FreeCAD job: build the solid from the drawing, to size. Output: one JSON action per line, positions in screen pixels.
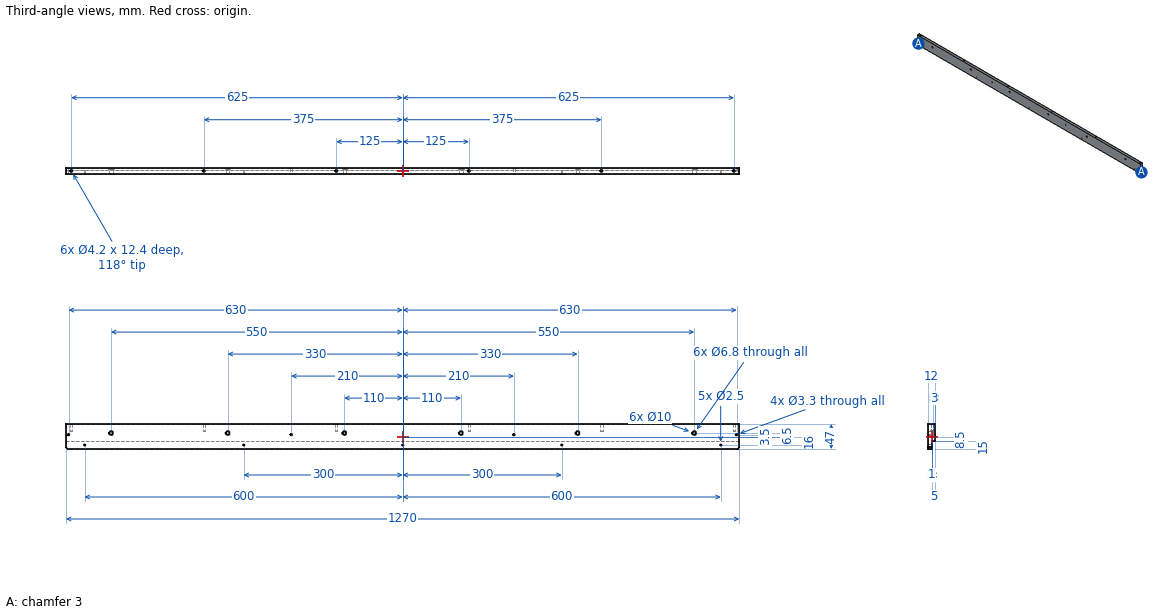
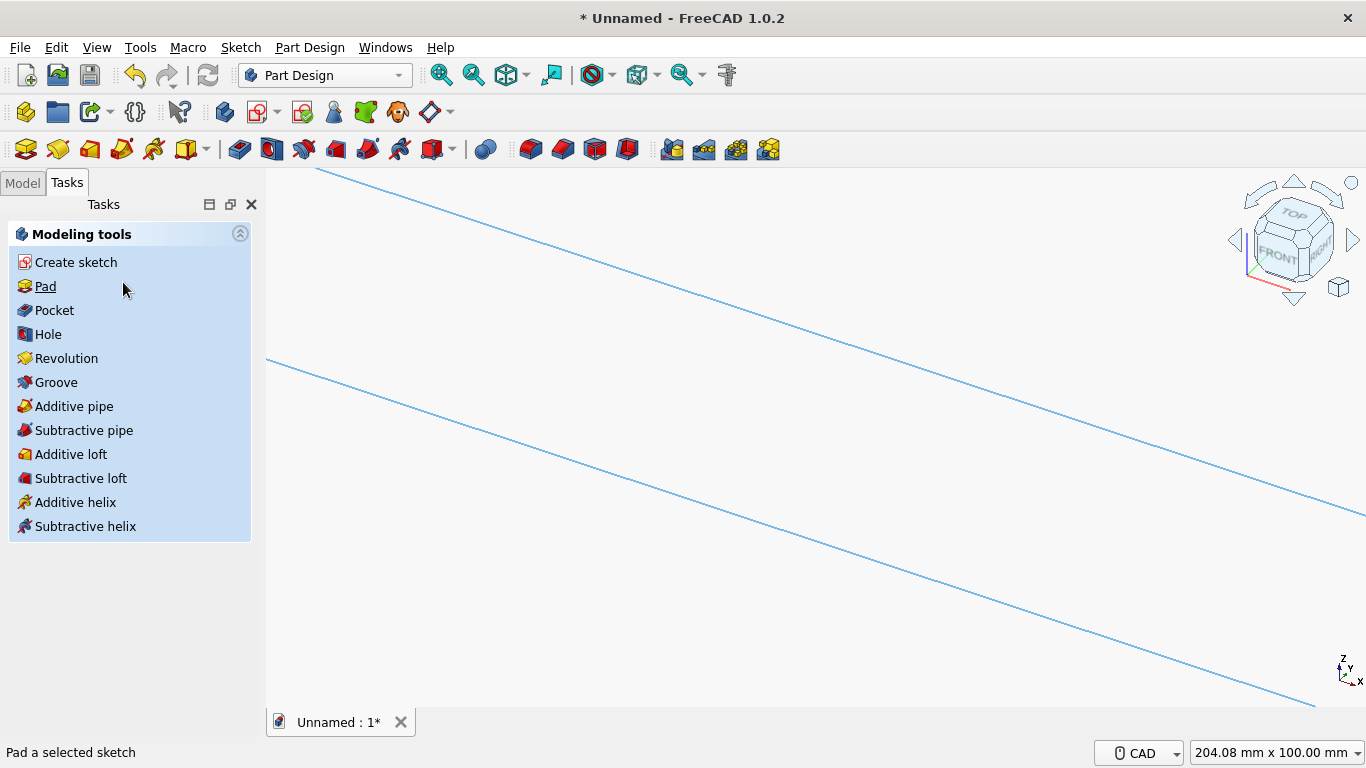
{"action": "left_click", "coordinate": [26, 150]}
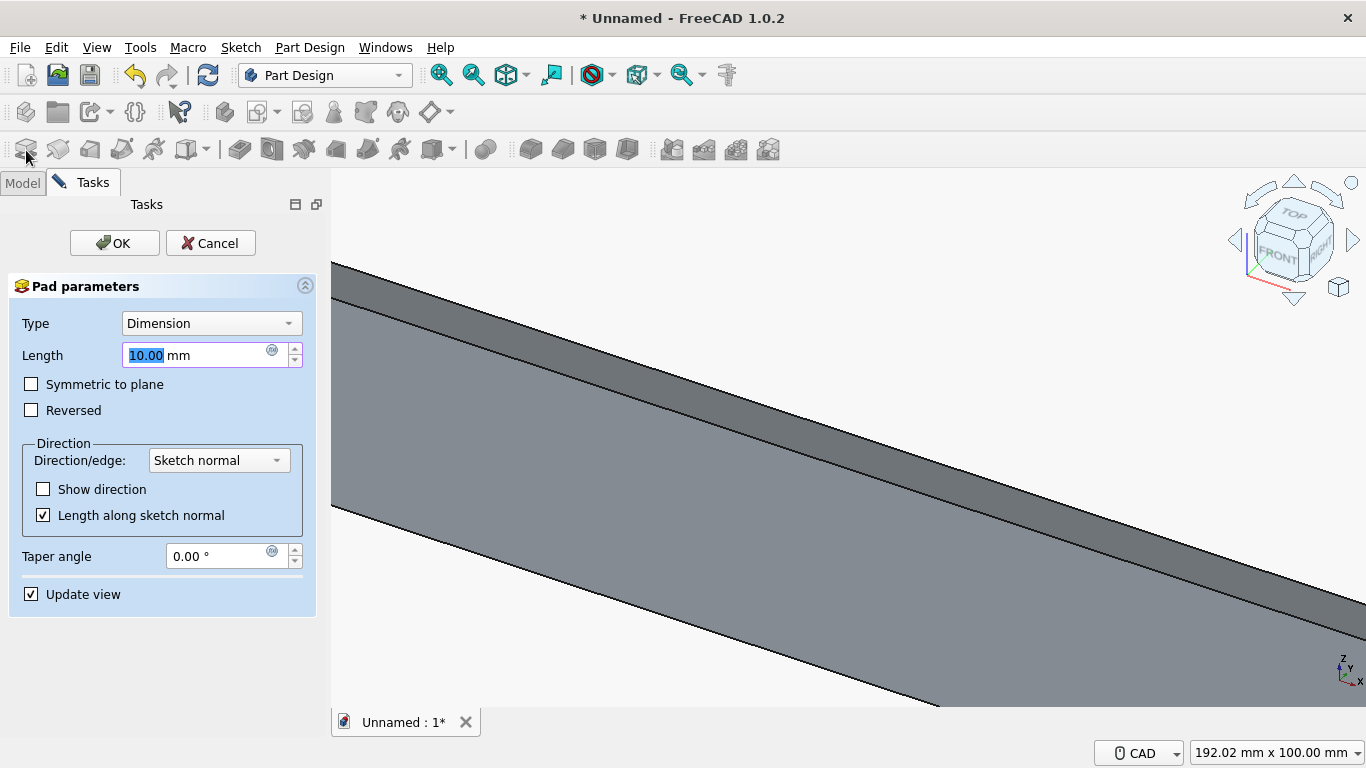
{"action": "type", "text": "12"}
{"action": "key", "text": "Tab"}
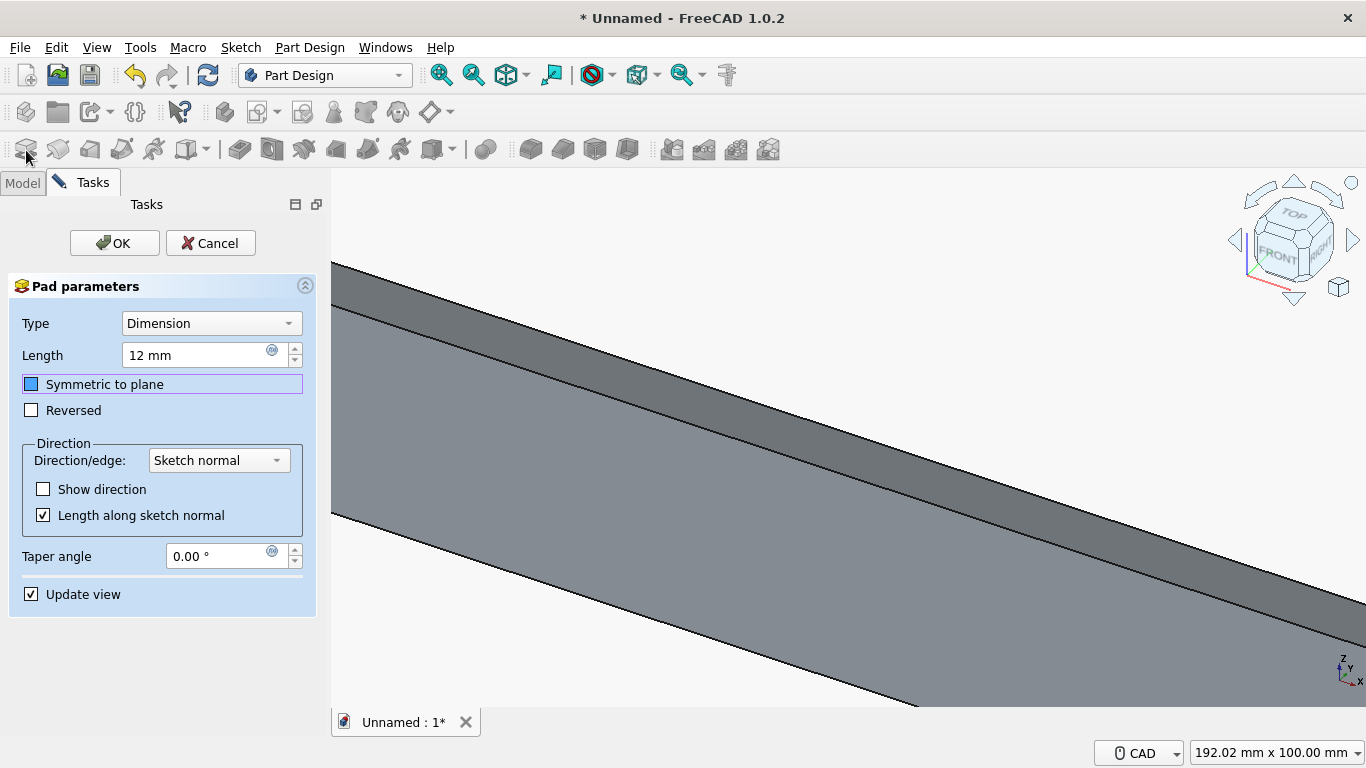
{"action": "left_click", "coordinate": [30, 384]}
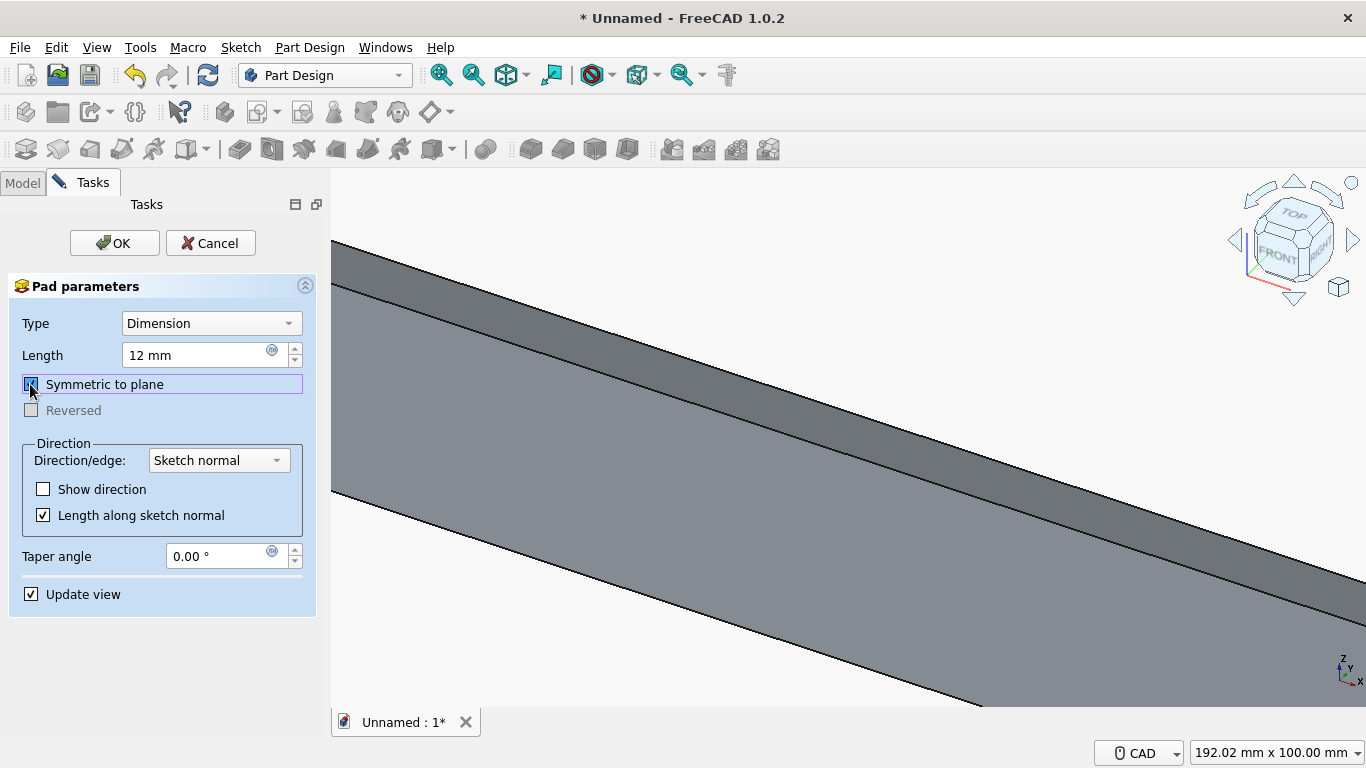
{"action": "left_click", "coordinate": [115, 243]}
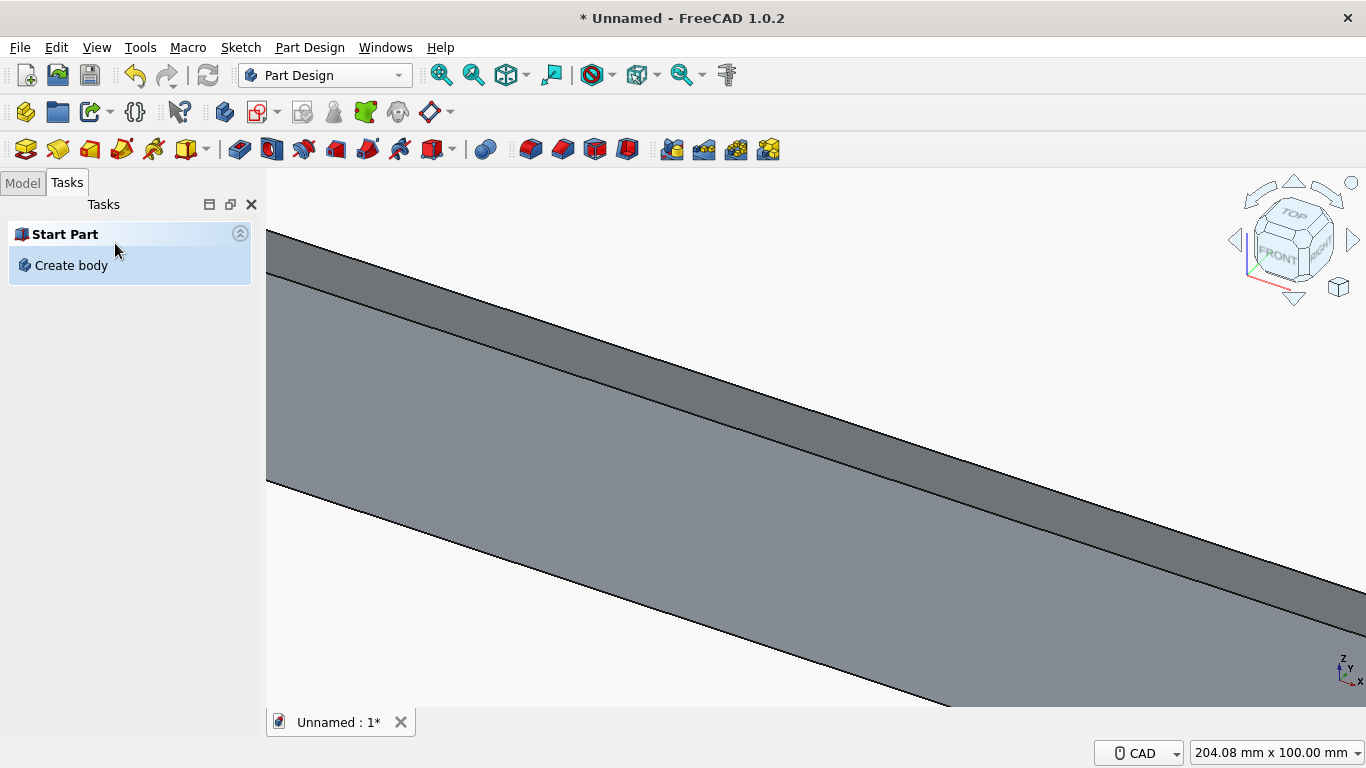
{"action": "key", "text": "v f"}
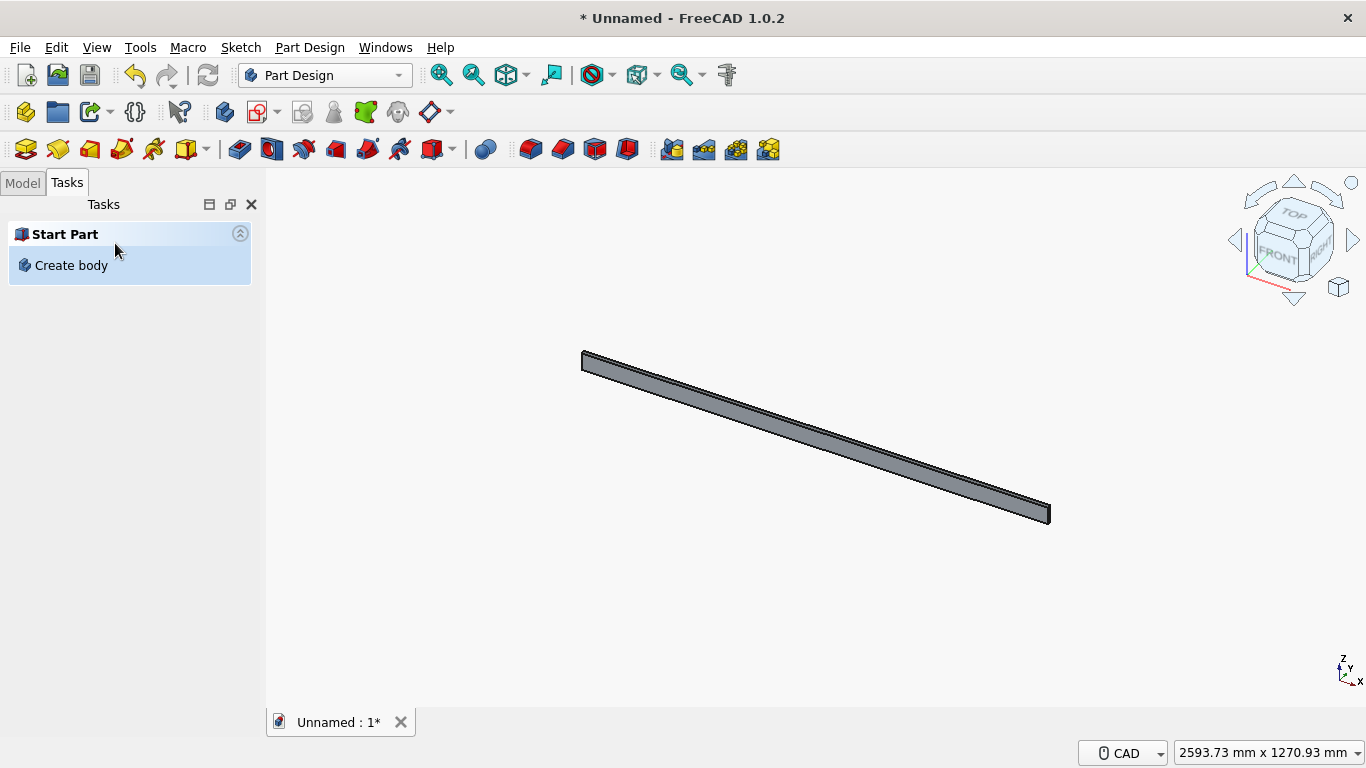
{"action": "scroll", "coordinate": [1049, 509], "scroll_direction": "up", "scroll_amount": 8}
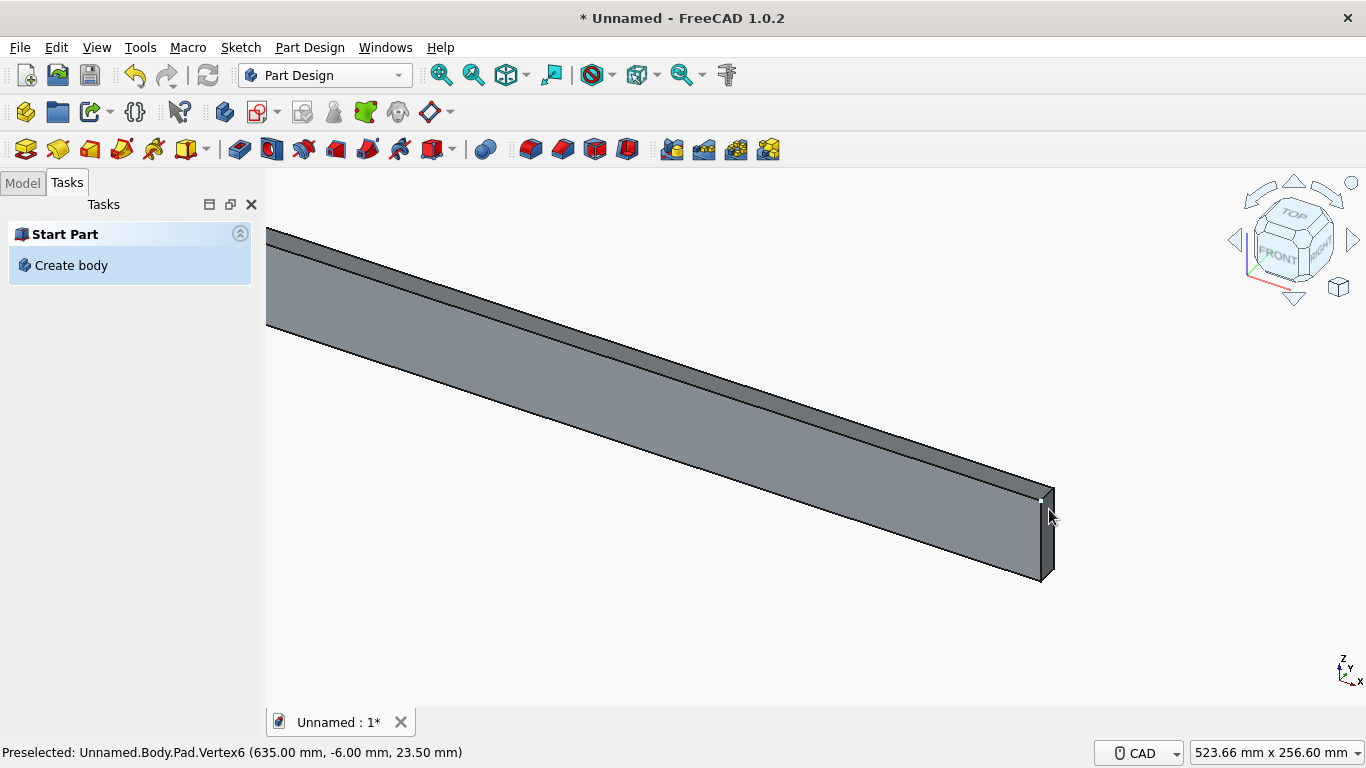
{"action": "left_click", "coordinate": [1049, 509]}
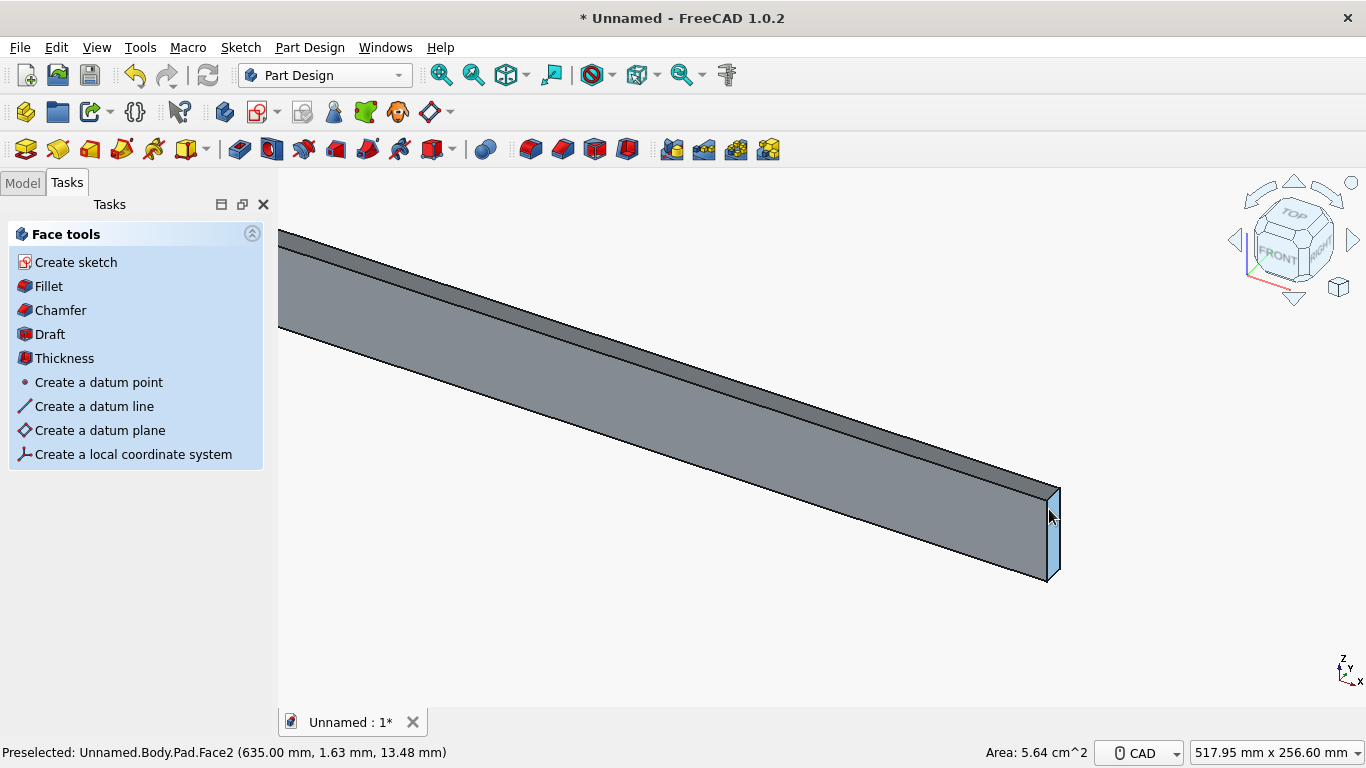
{"action": "left_click", "coordinate": [258, 112]}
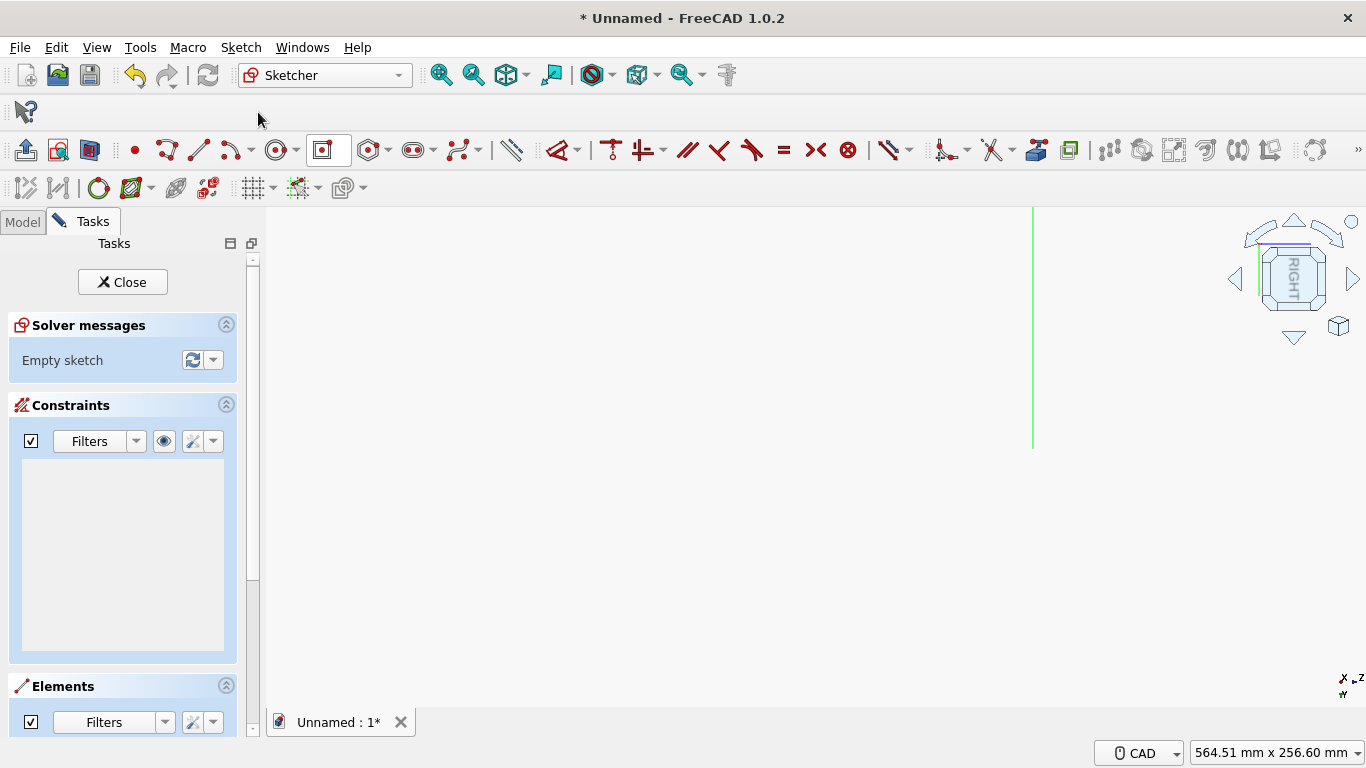
{"action": "scroll", "coordinate": [748, 457], "scroll_direction": "down", "scroll_amount": 5}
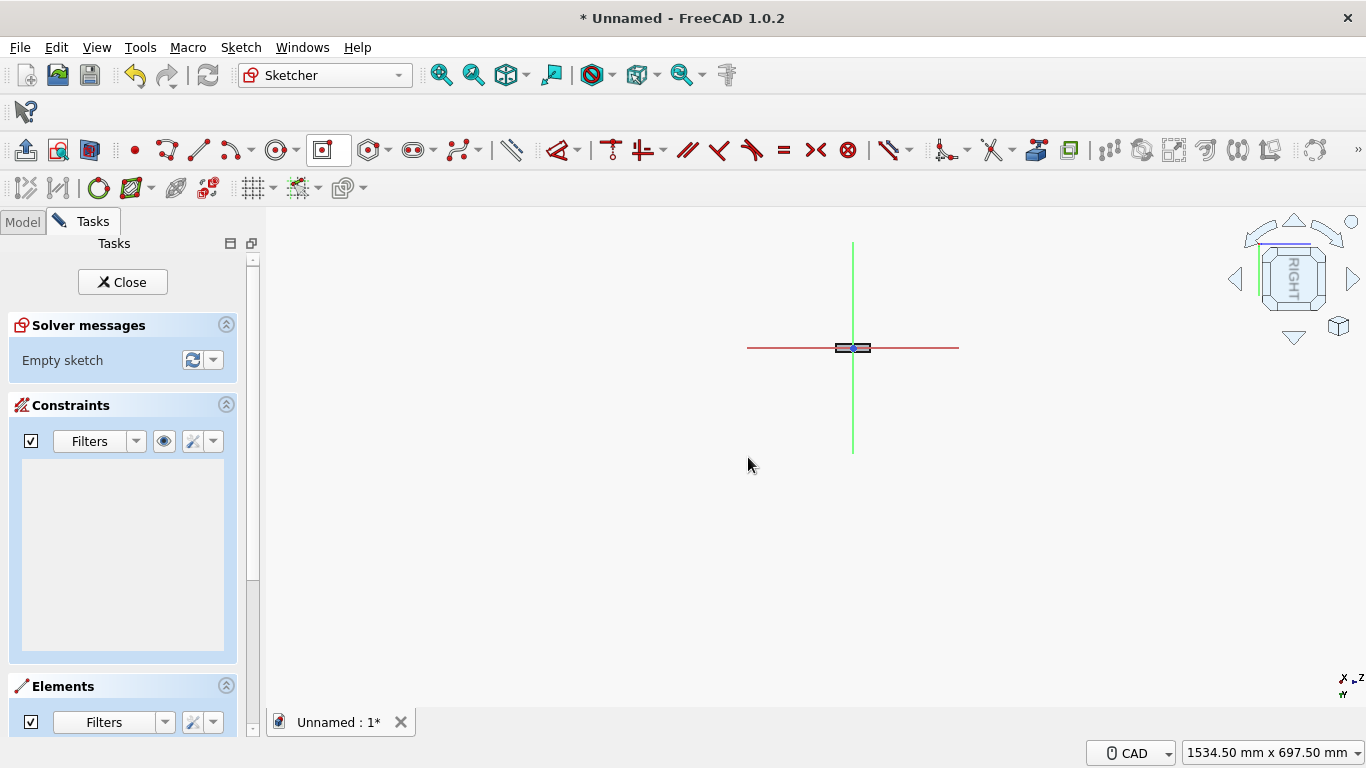
{"action": "scroll", "coordinate": [850, 345], "scroll_direction": "up", "scroll_amount": 15}